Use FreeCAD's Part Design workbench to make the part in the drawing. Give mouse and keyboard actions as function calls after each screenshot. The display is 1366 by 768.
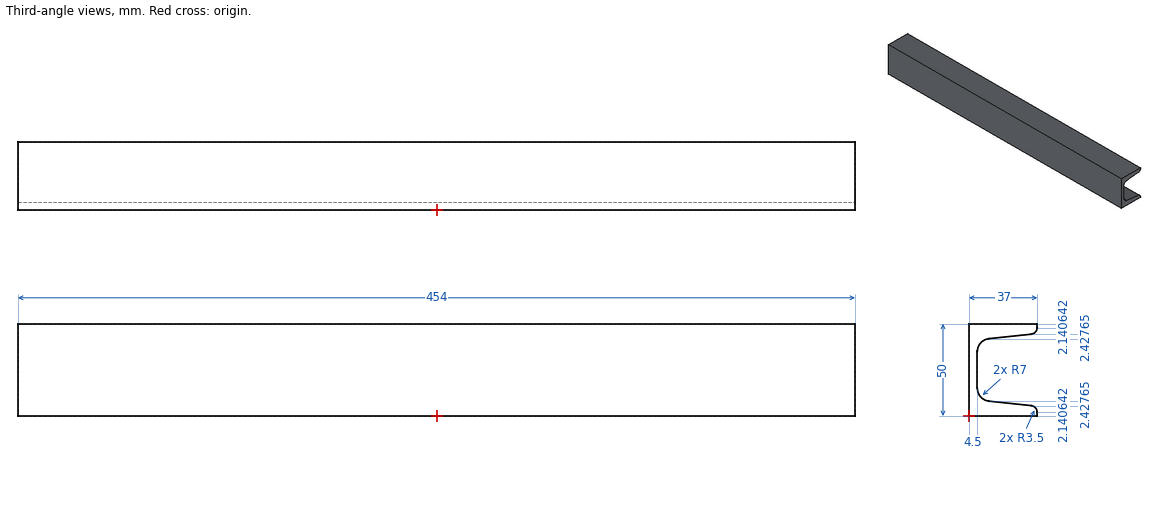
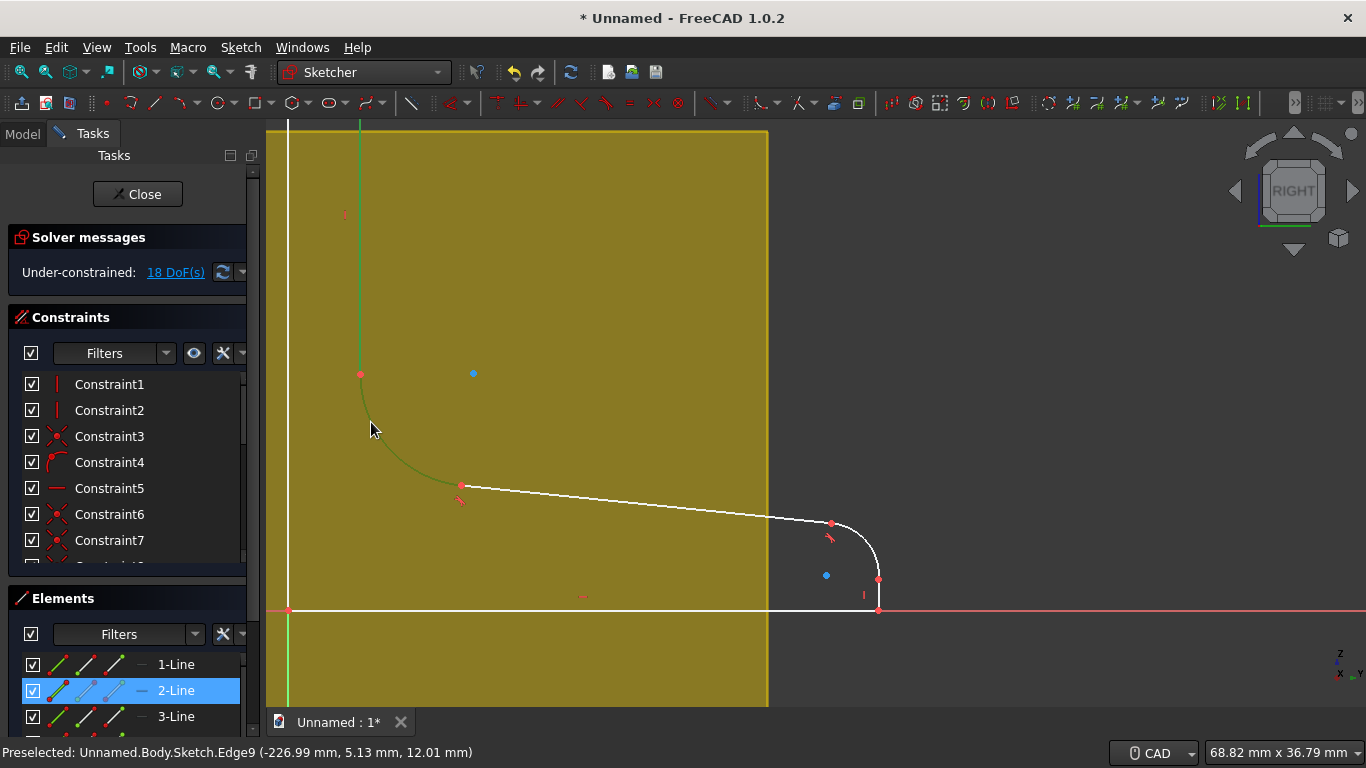
click(606, 104)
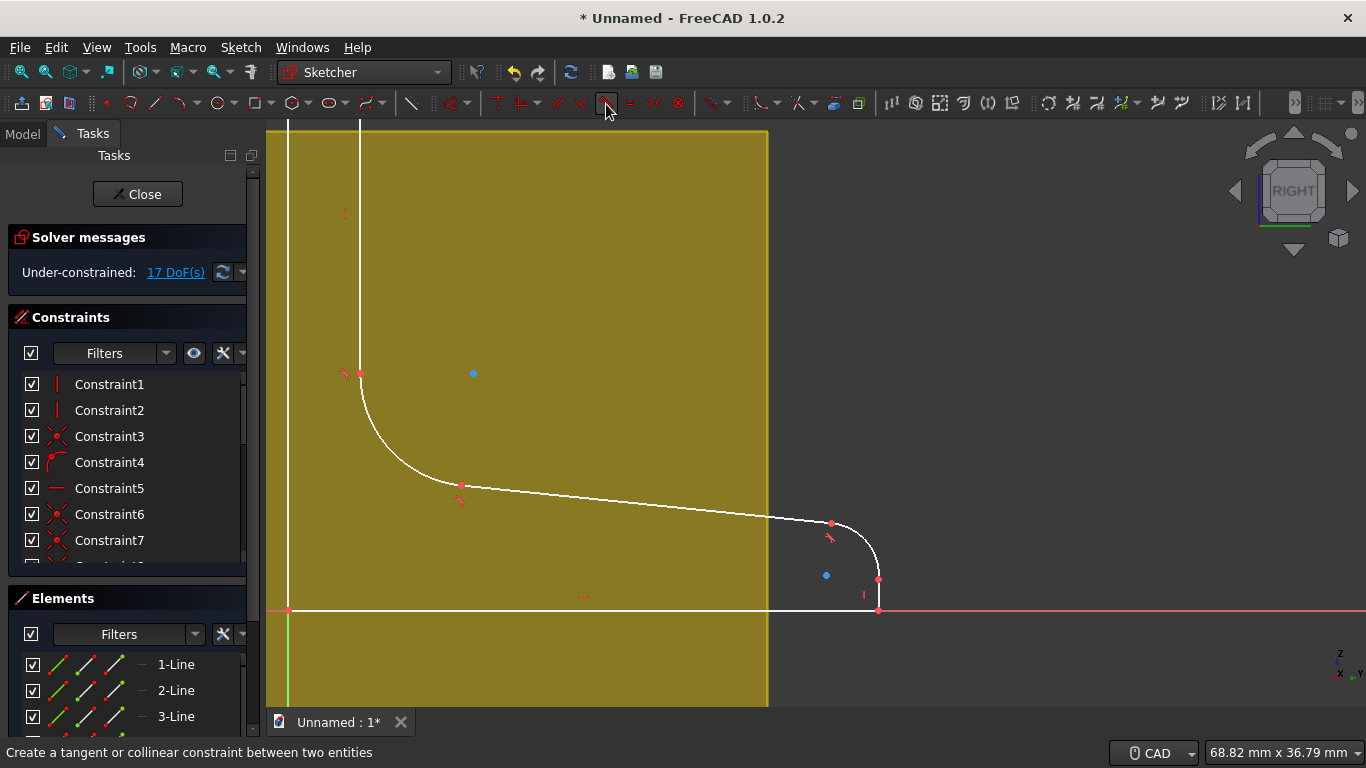
click(360, 278)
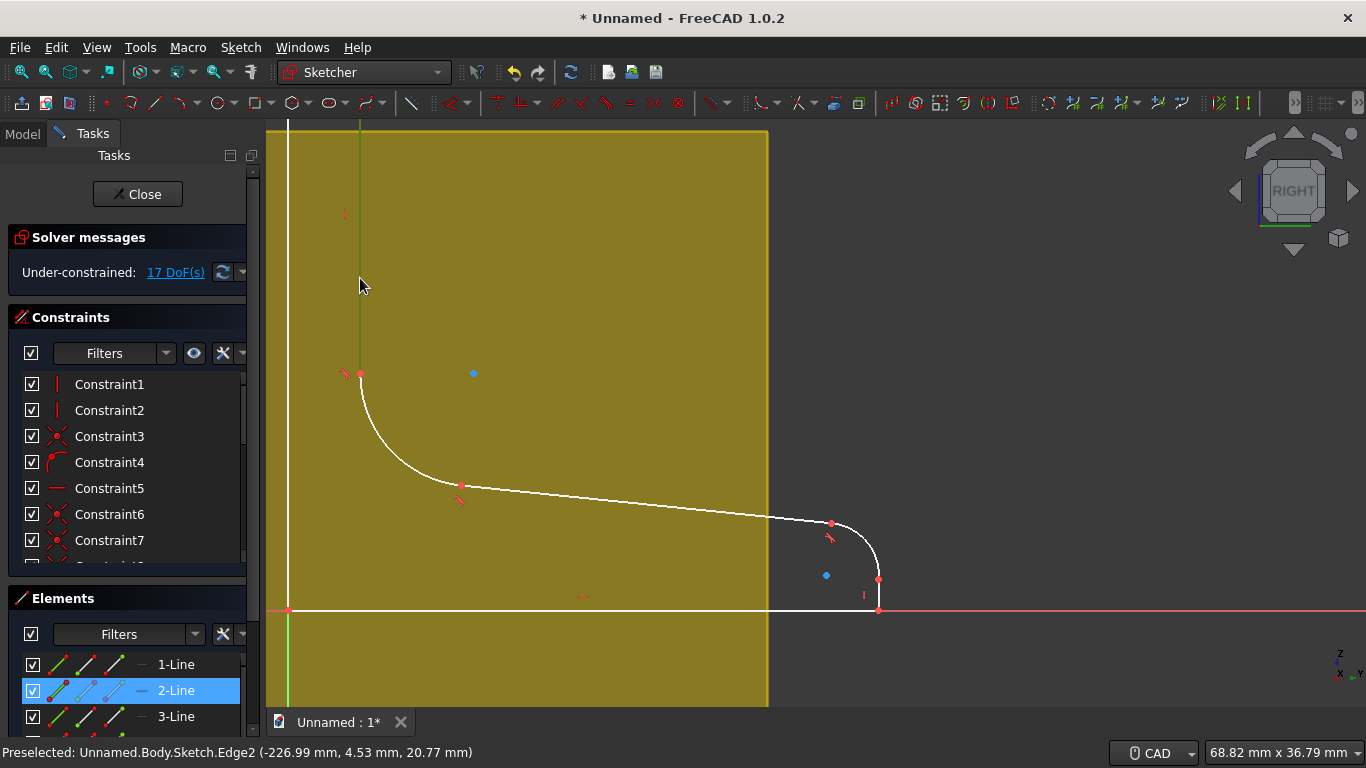
scroll(881, 578, down, 4)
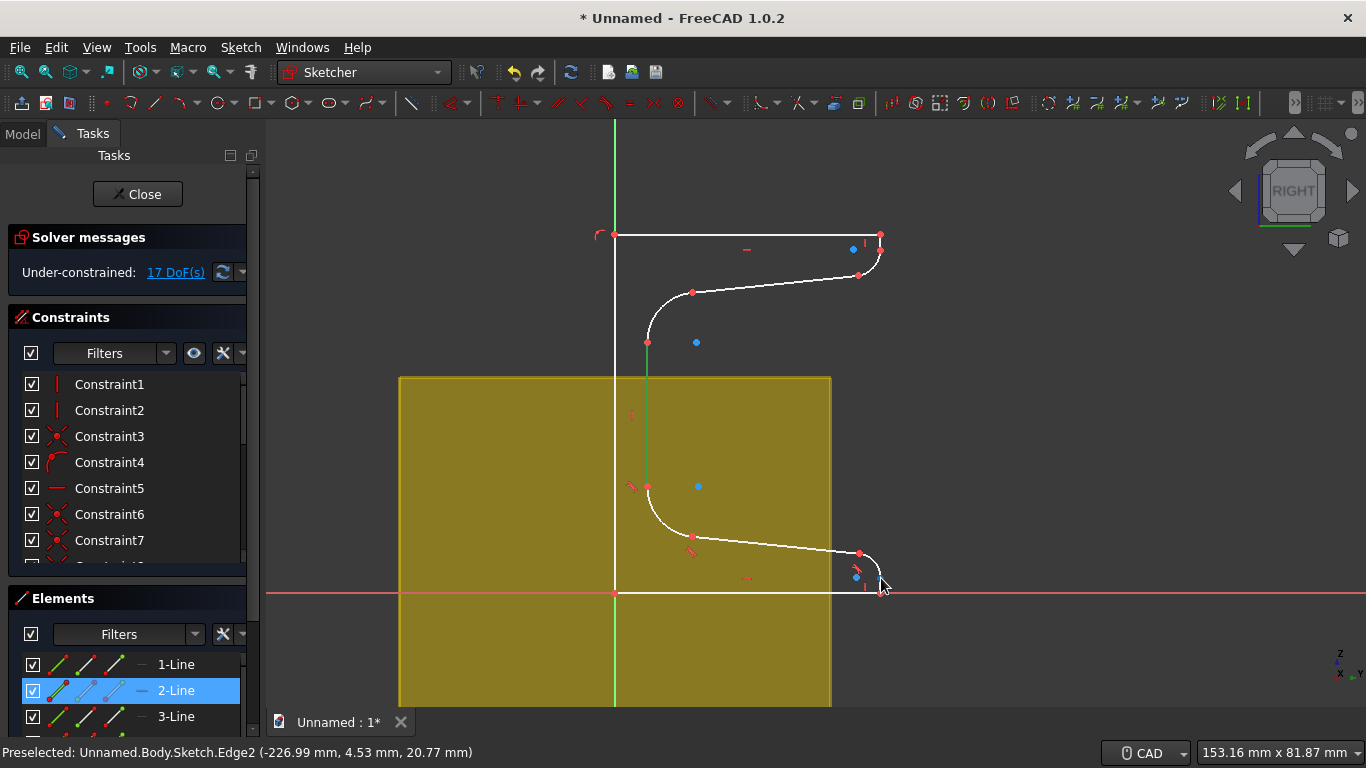
click(671, 300)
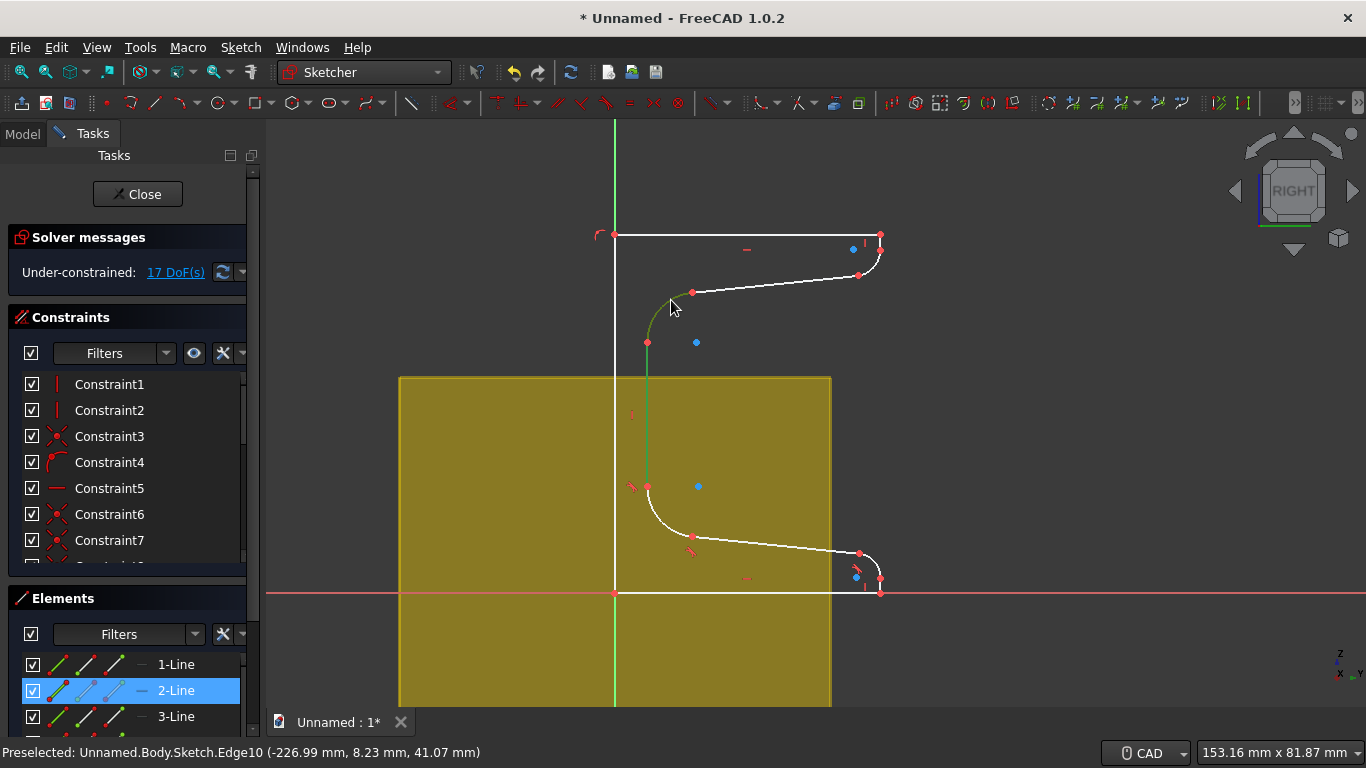
key(t)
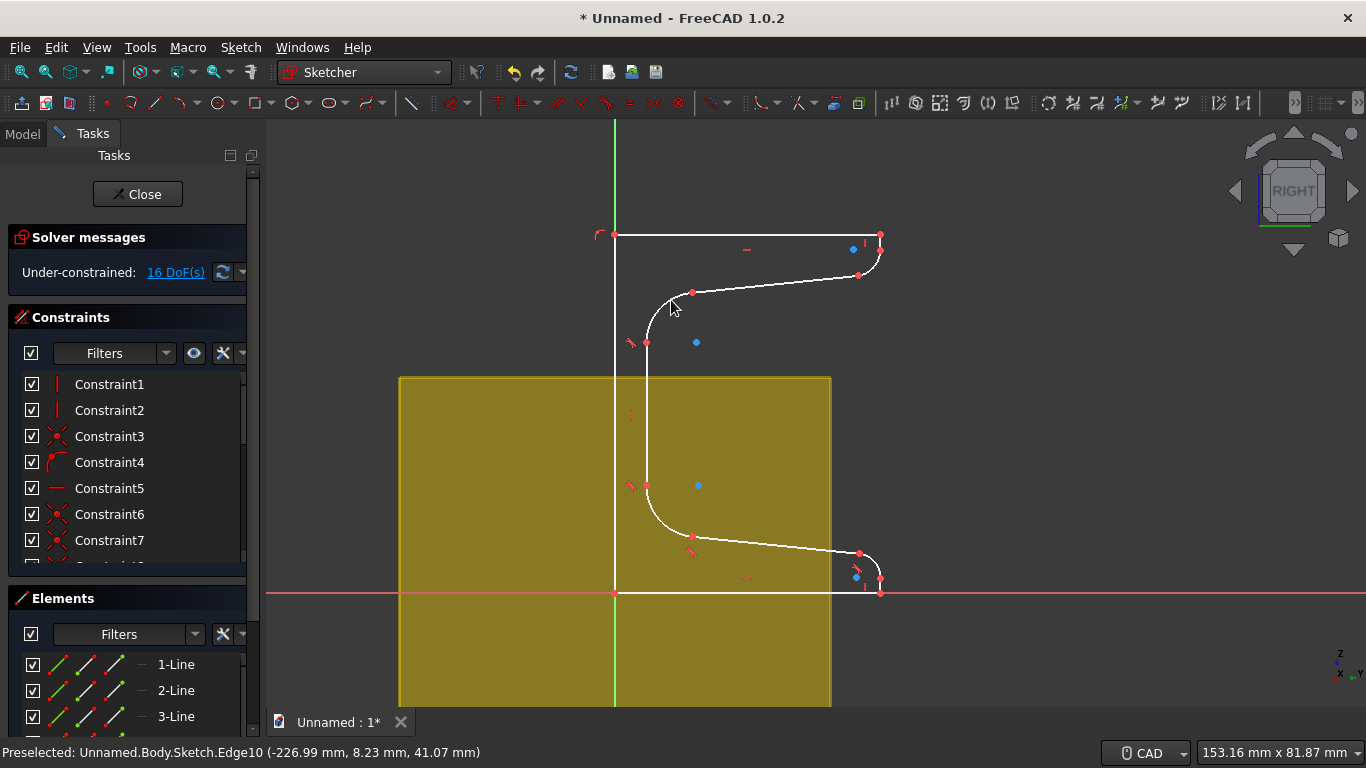
click(742, 288)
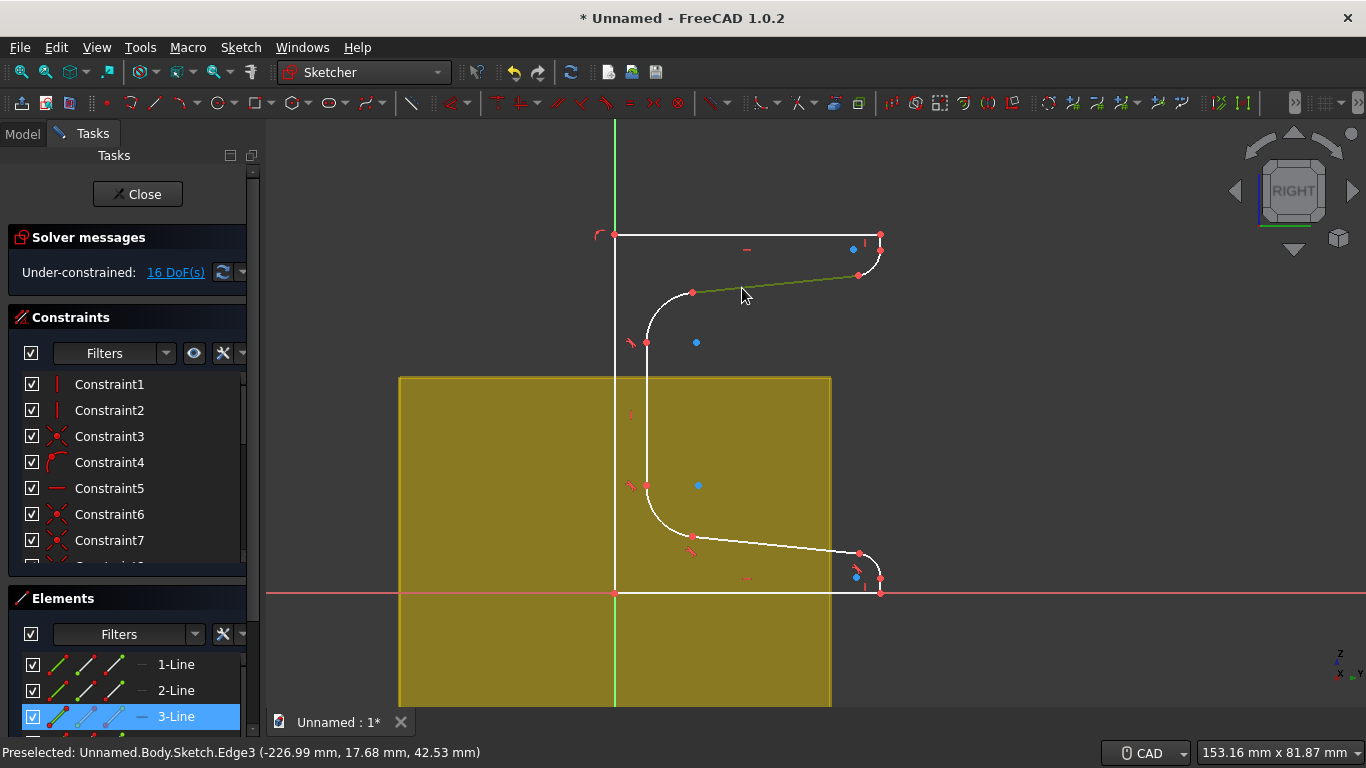
click(671, 300)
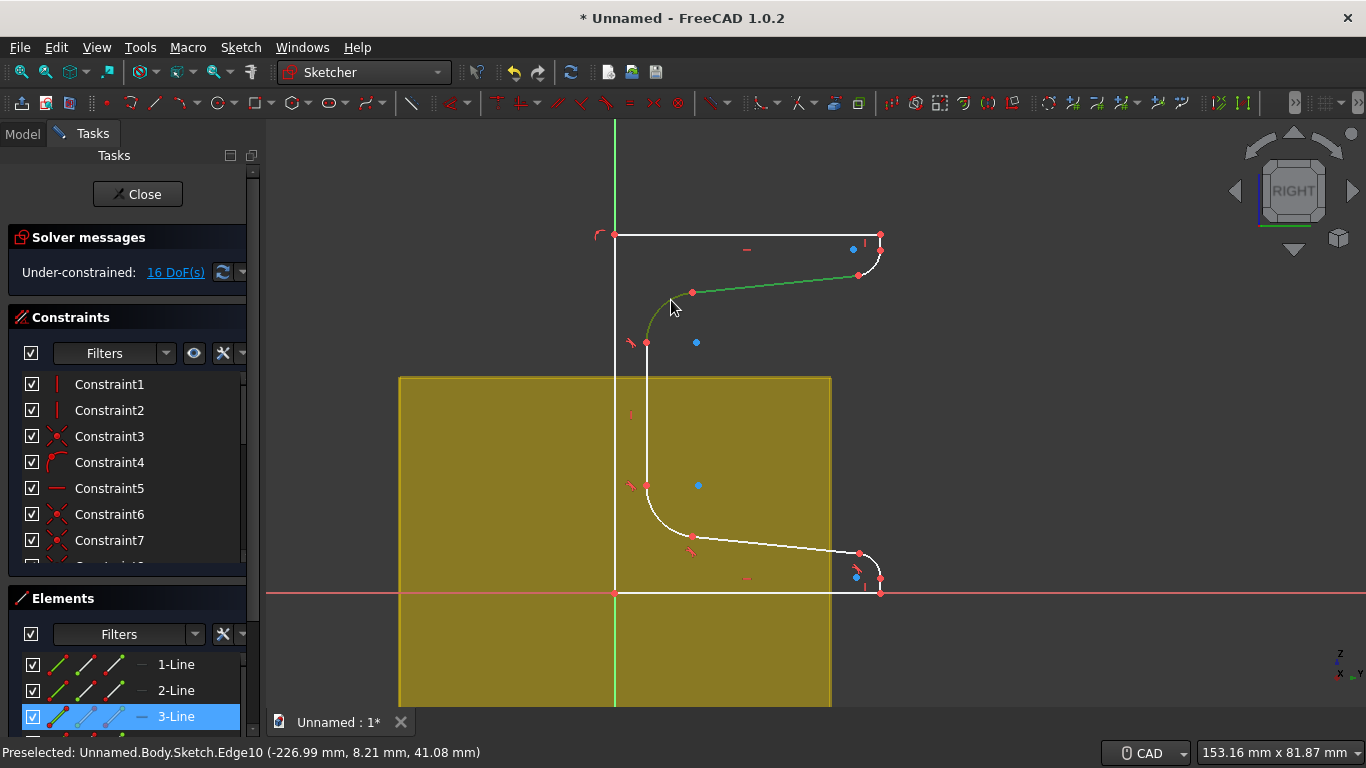
click(606, 104)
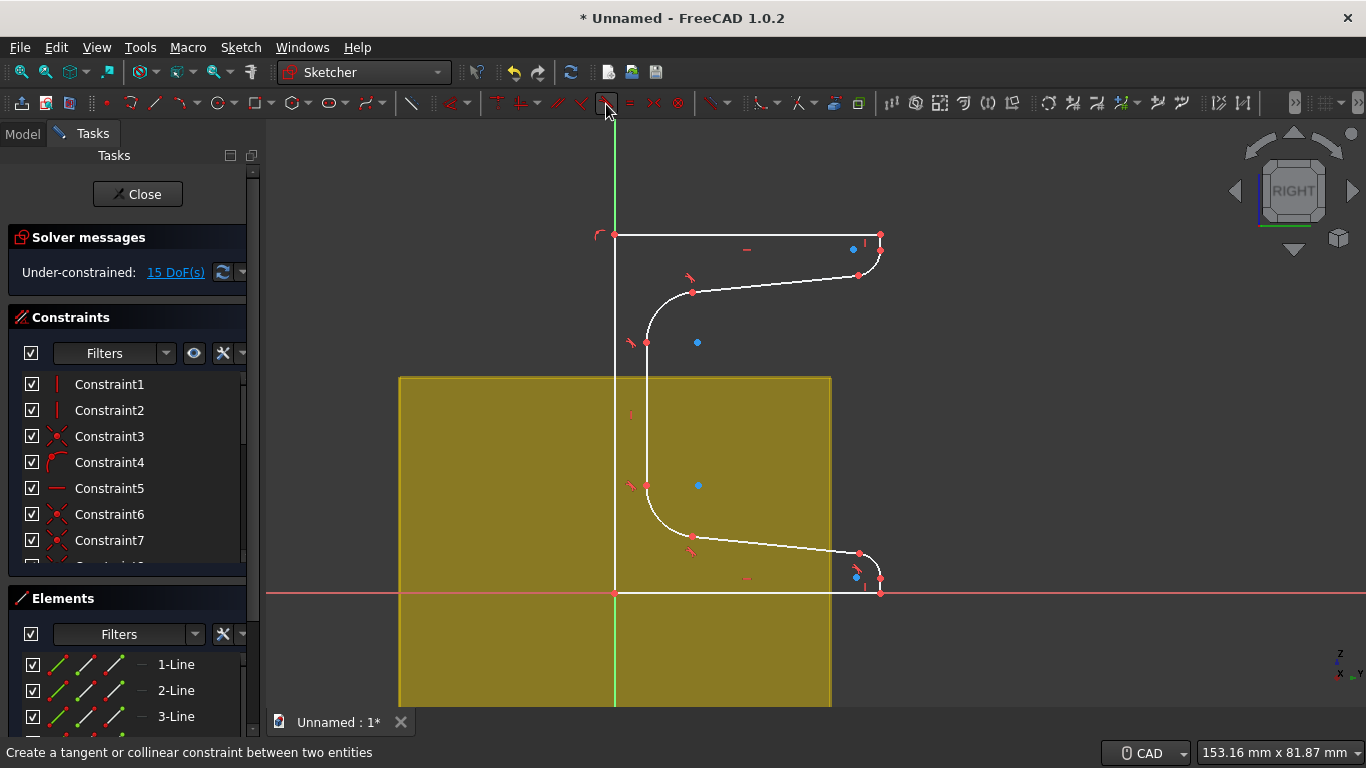
click(742, 287)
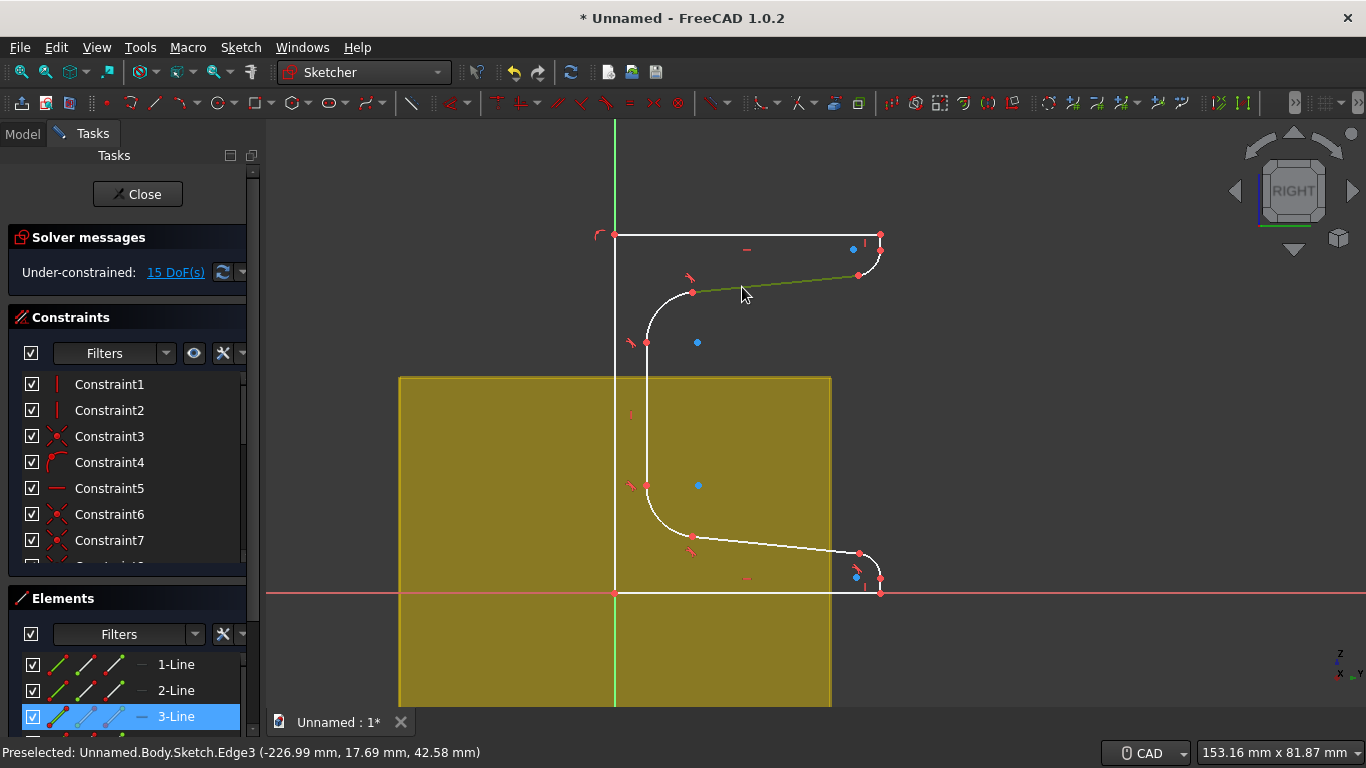
scroll(868, 272, up, 2)